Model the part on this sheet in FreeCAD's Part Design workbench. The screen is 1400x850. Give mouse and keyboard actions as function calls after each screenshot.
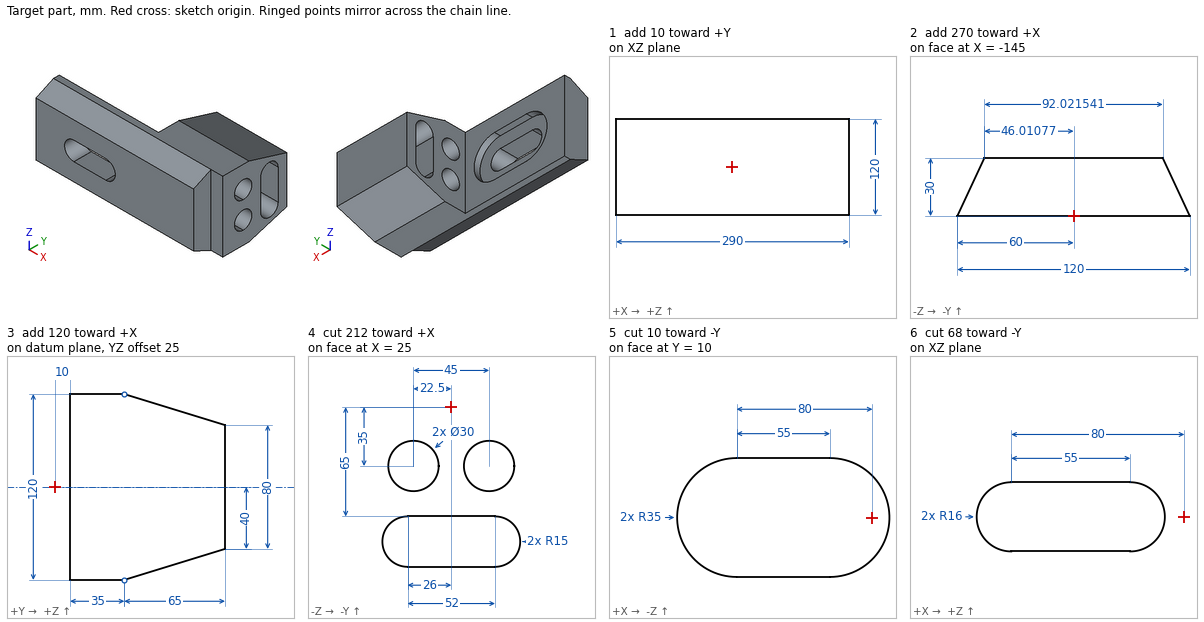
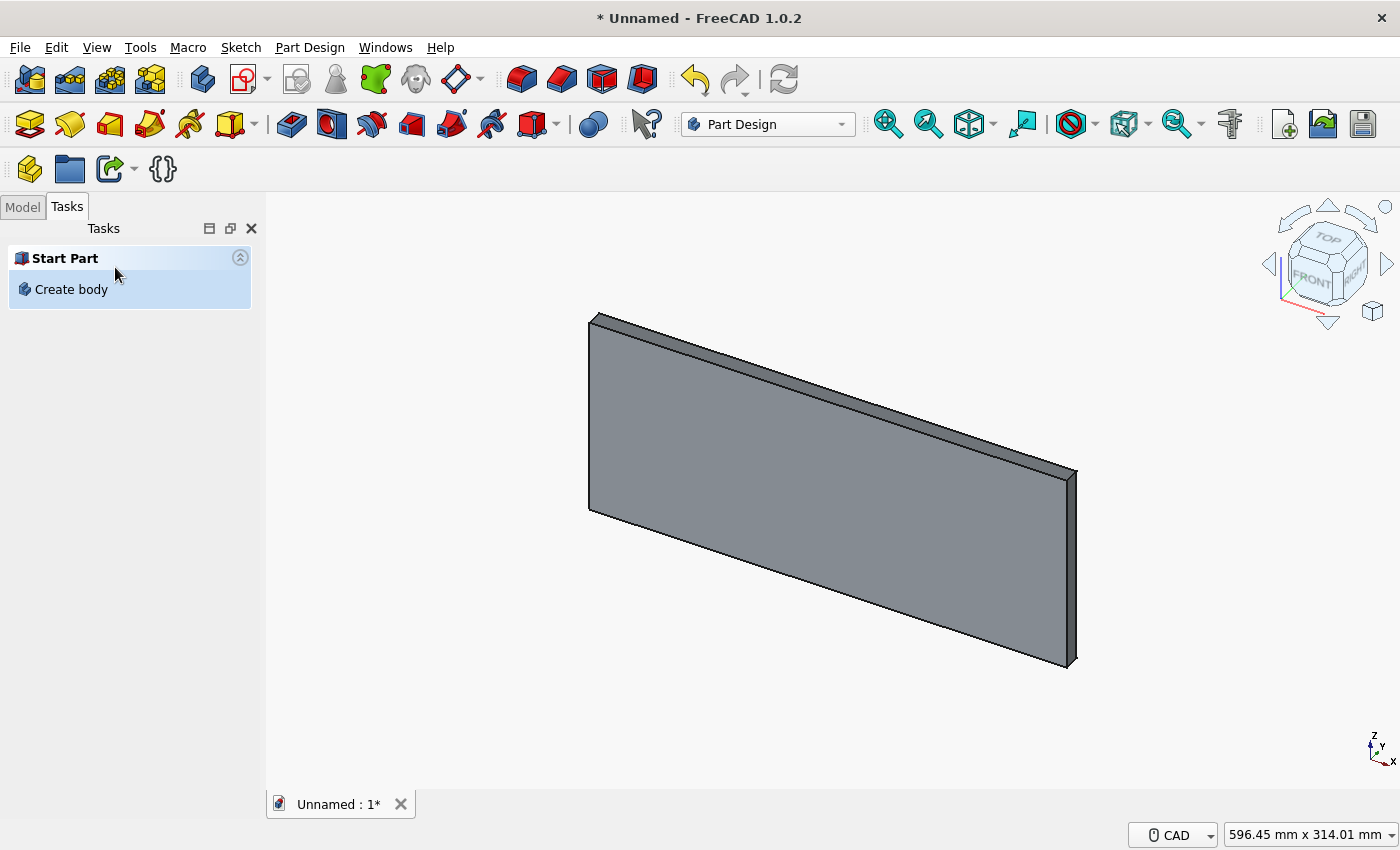
key(6)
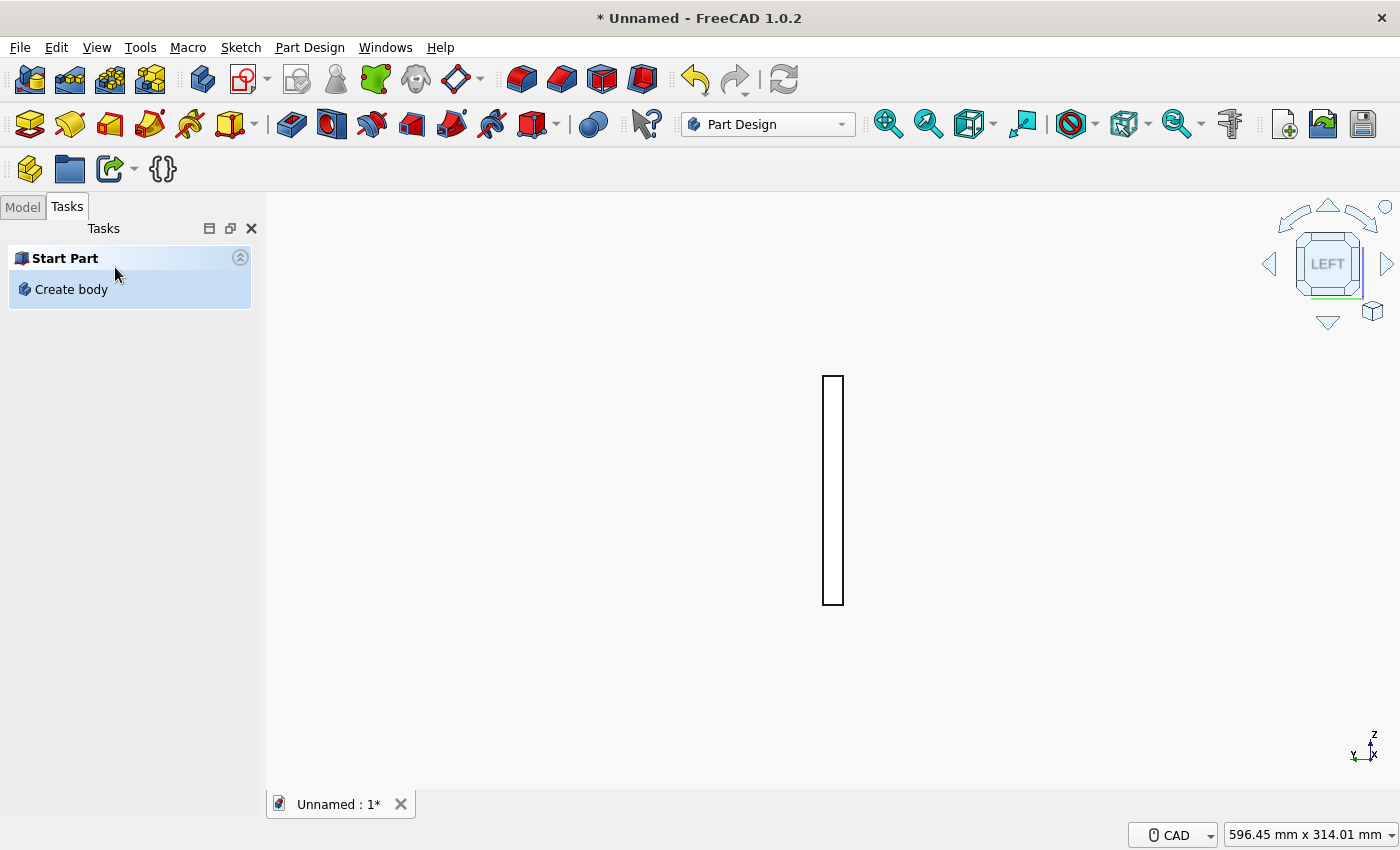
click(890, 124)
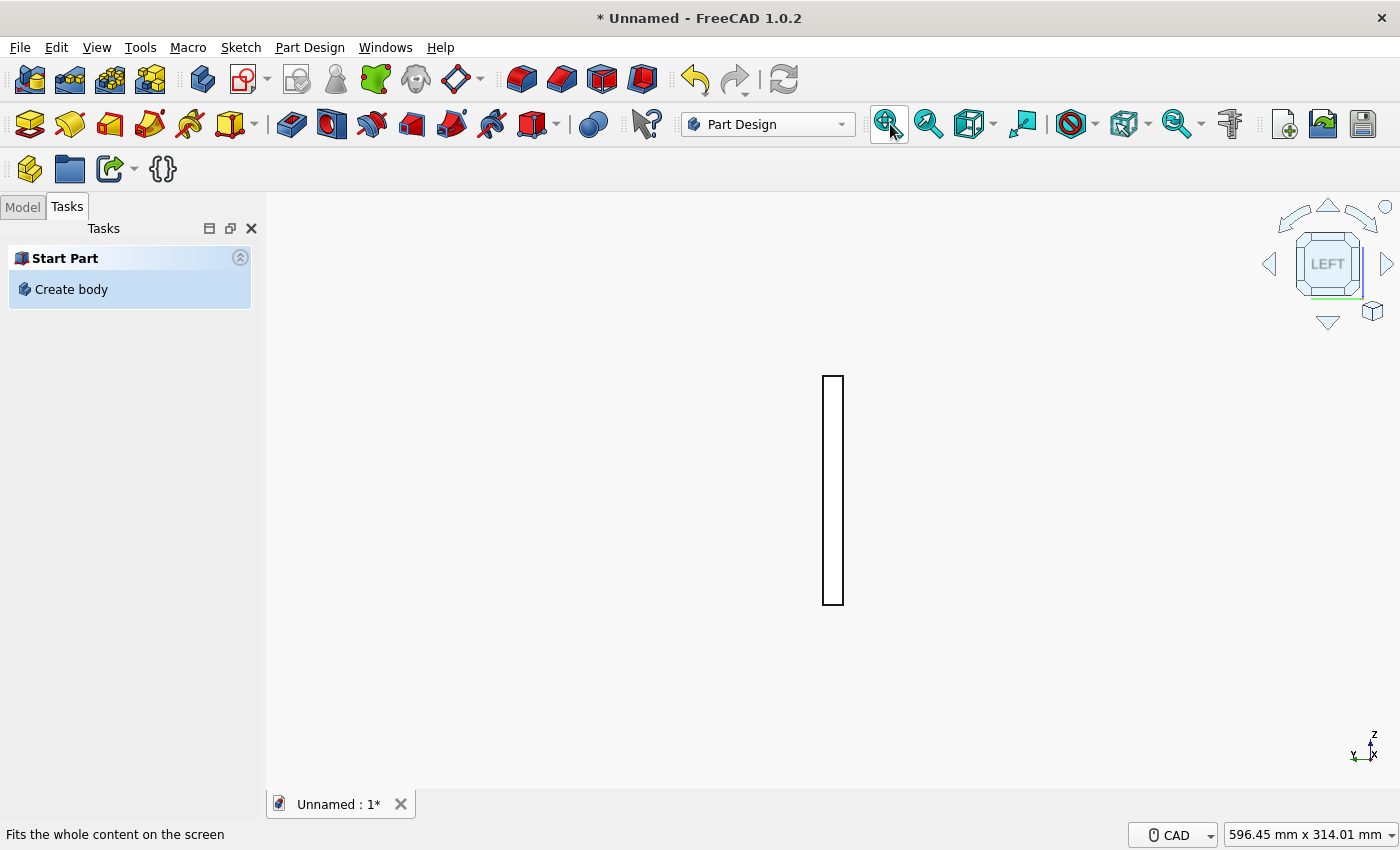
click(833, 457)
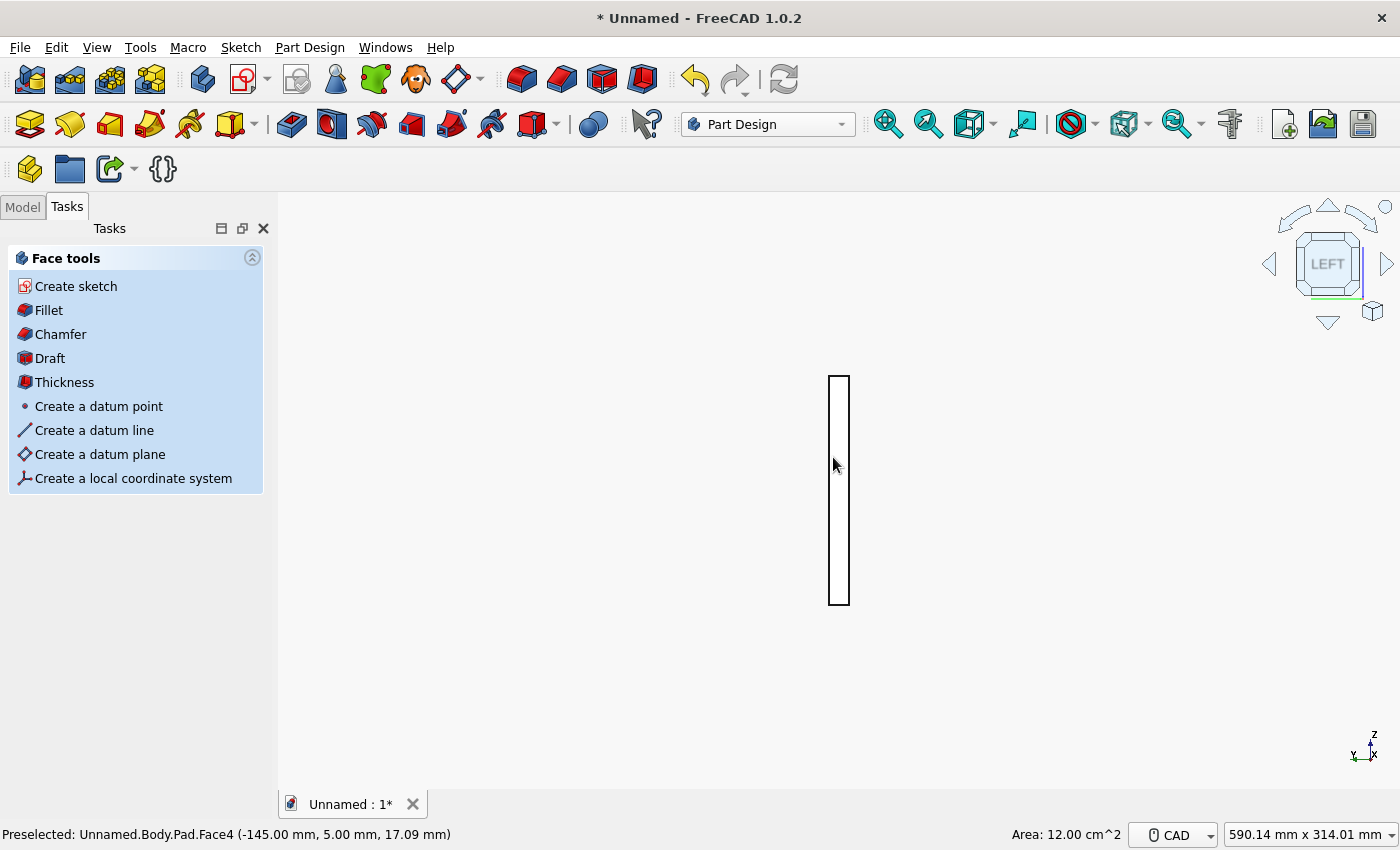
click(244, 80)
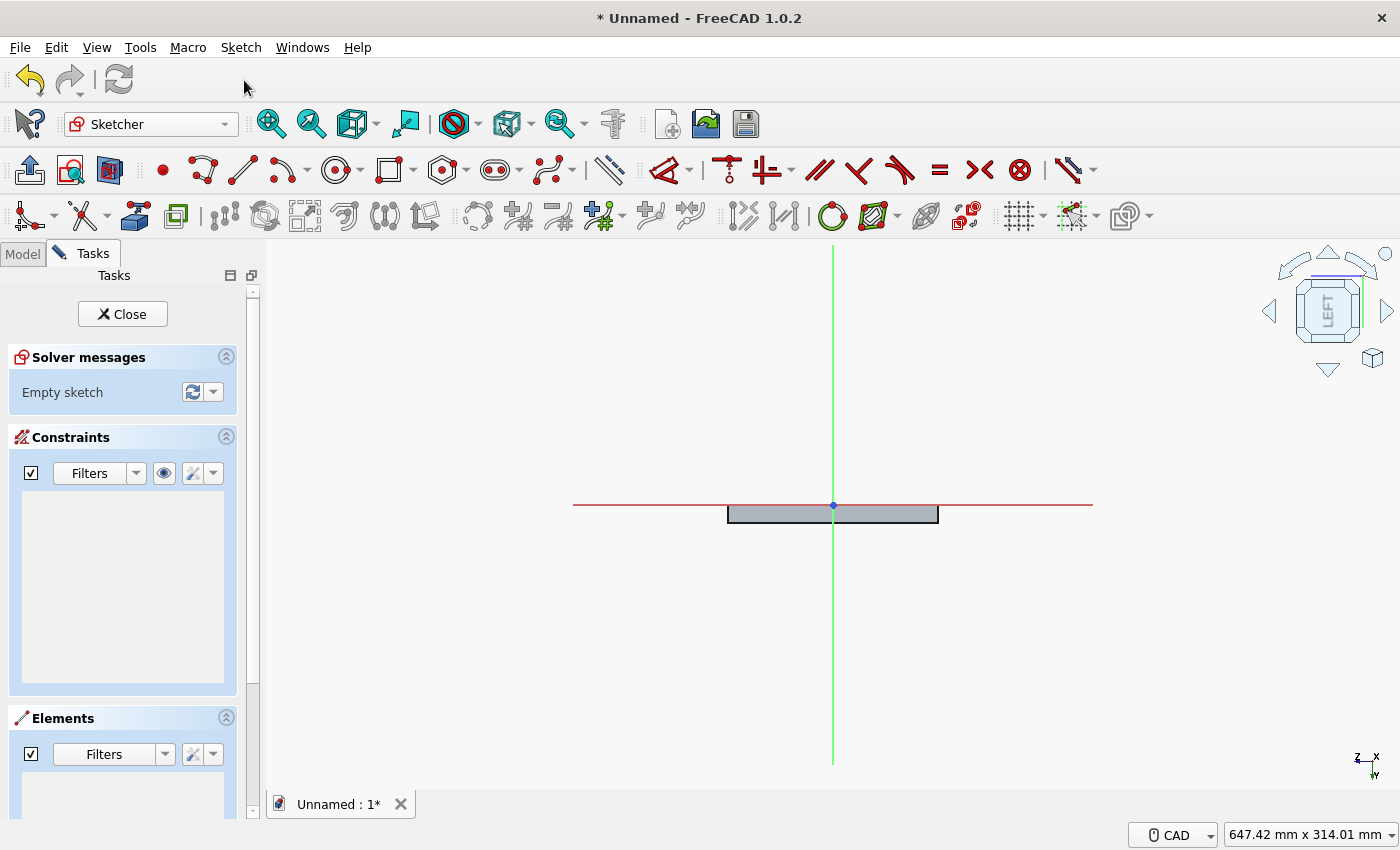
scroll(863, 464, up, 6)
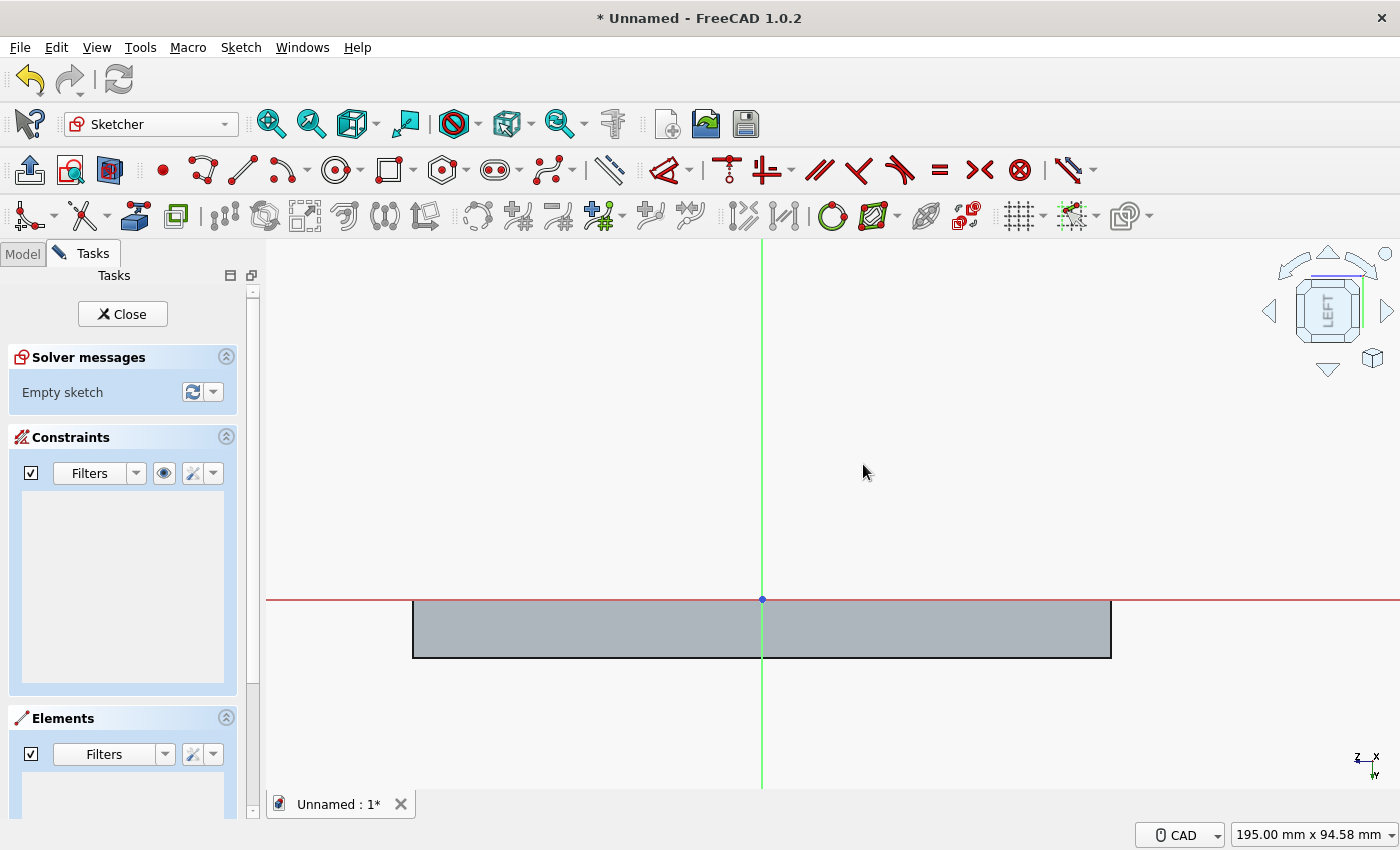
key(g)
key(m)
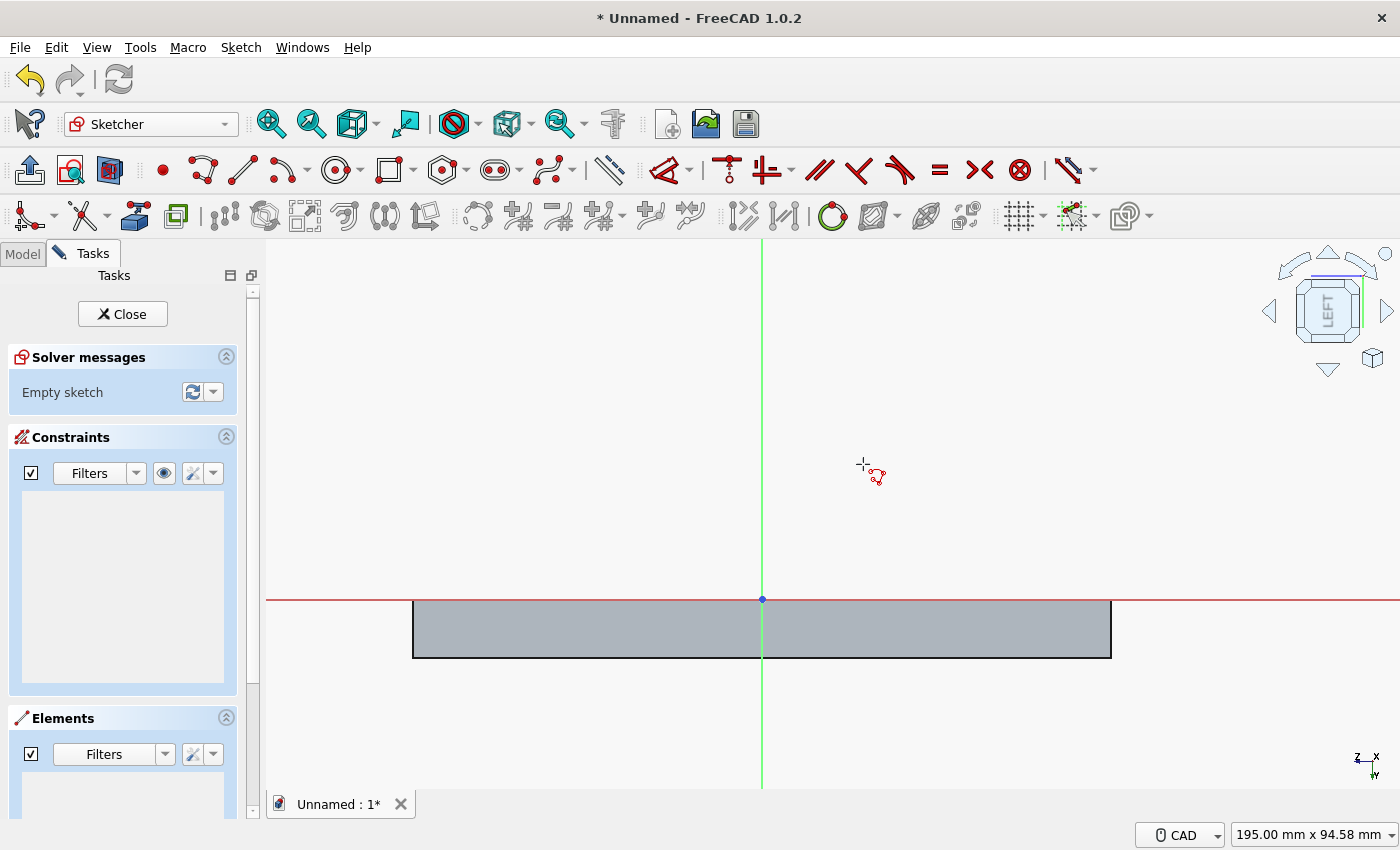
click(495, 426)
click(413, 600)
click(1111, 591)
click(1030, 426)
click(495, 427)
key(Escape)
key(Escape)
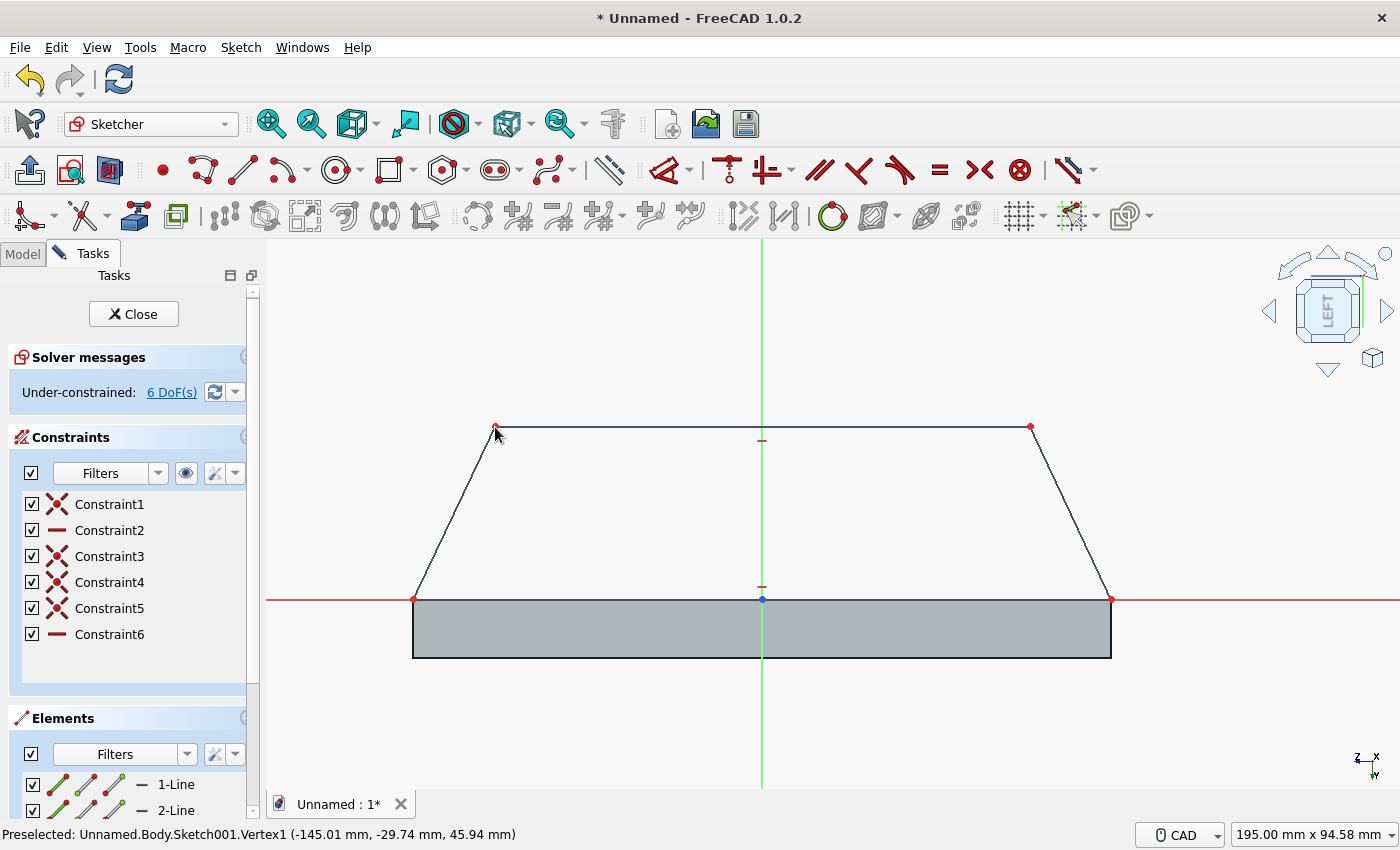
click(413, 600)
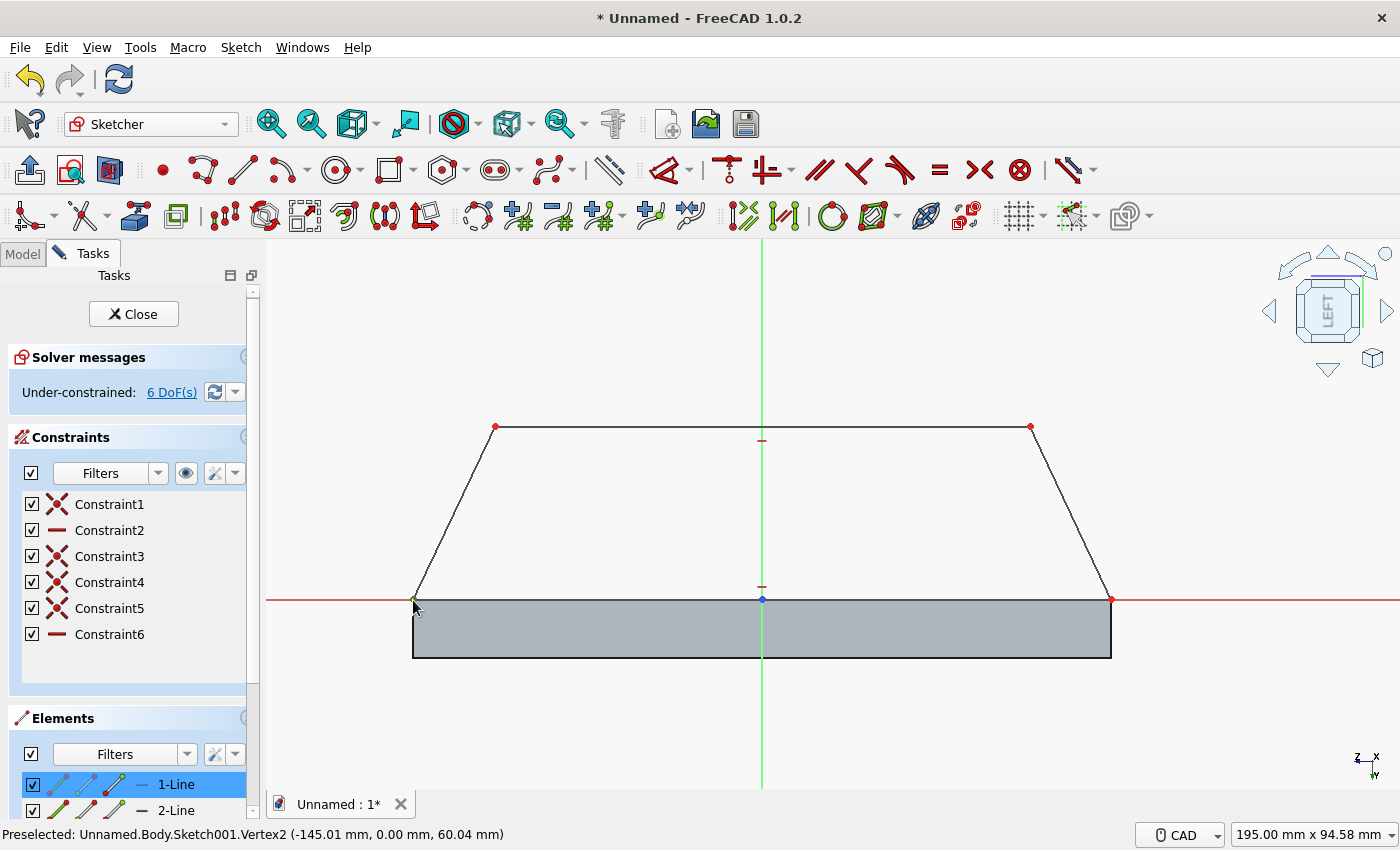
click(361, 600)